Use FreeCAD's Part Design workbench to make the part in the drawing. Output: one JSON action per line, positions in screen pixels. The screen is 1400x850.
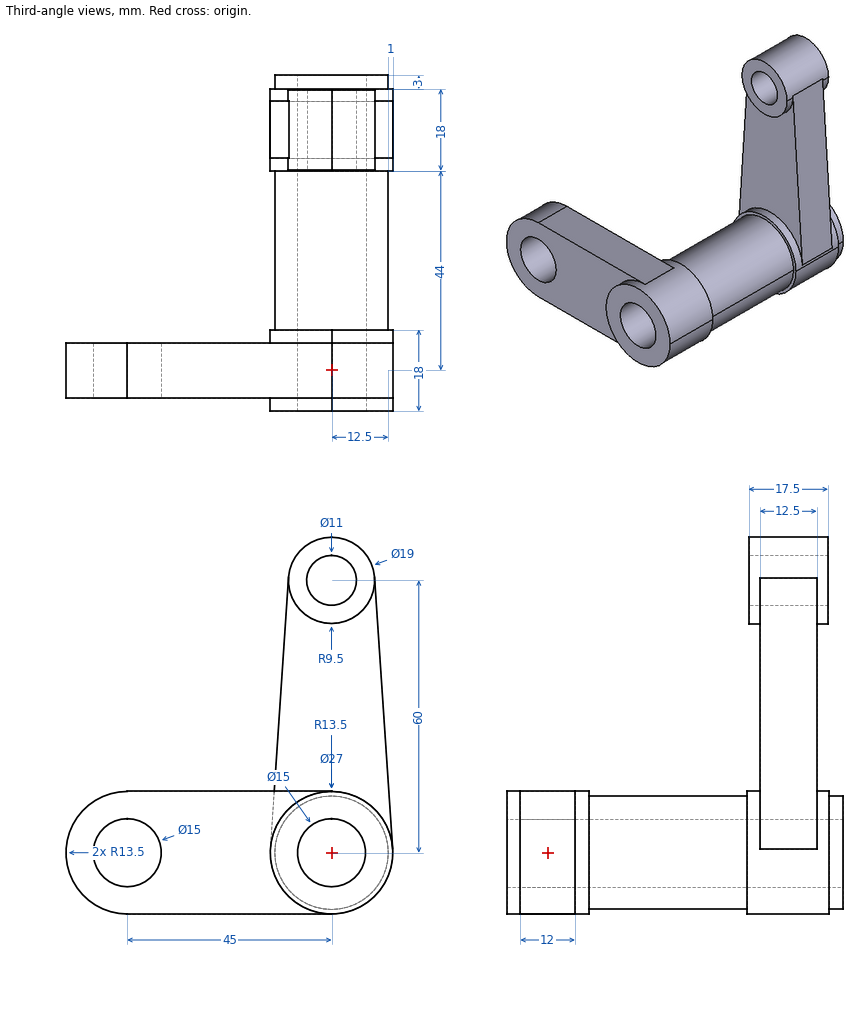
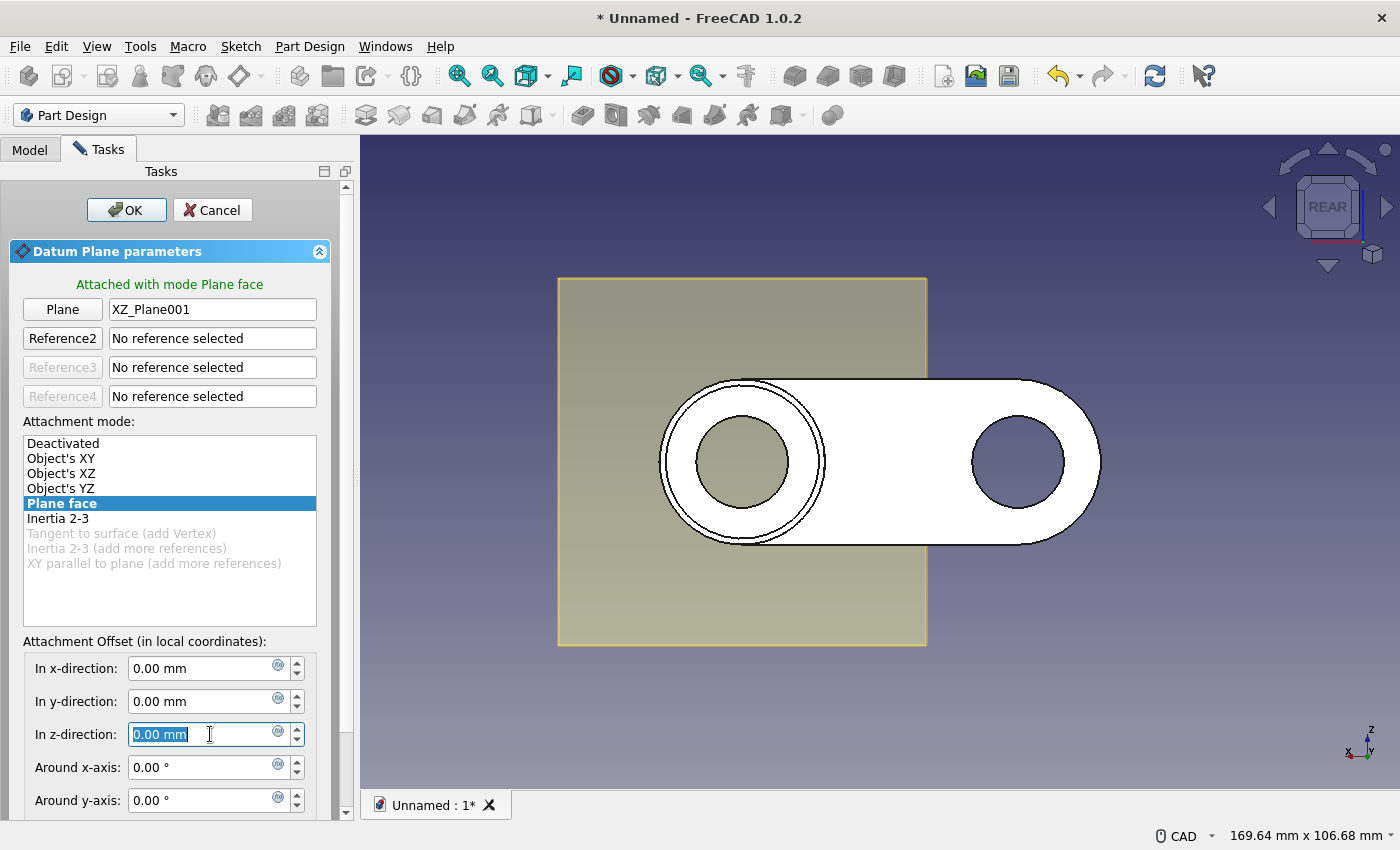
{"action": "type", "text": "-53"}
{"action": "key", "text": "Tab"}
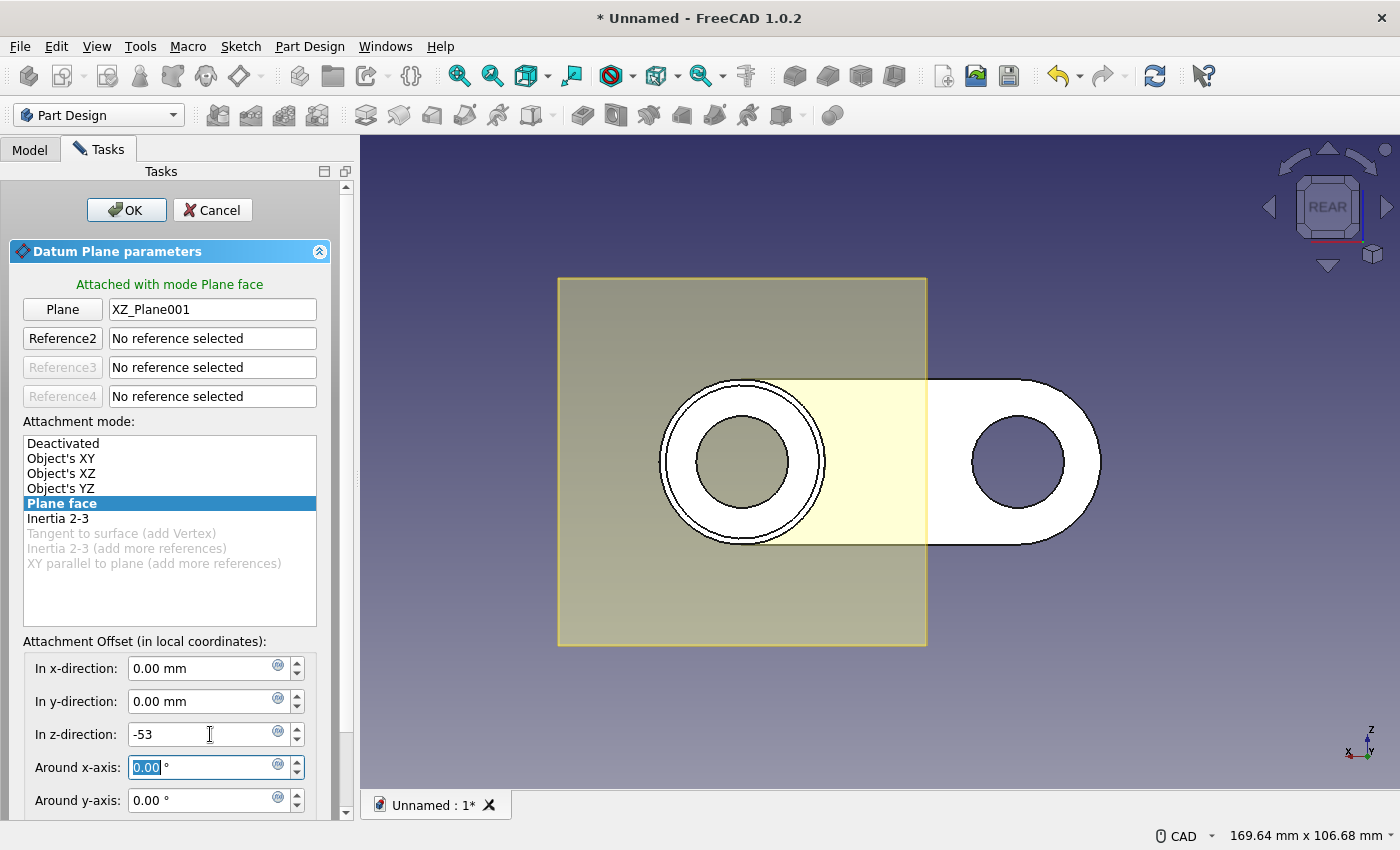
{"action": "left_click", "coordinate": [127, 210]}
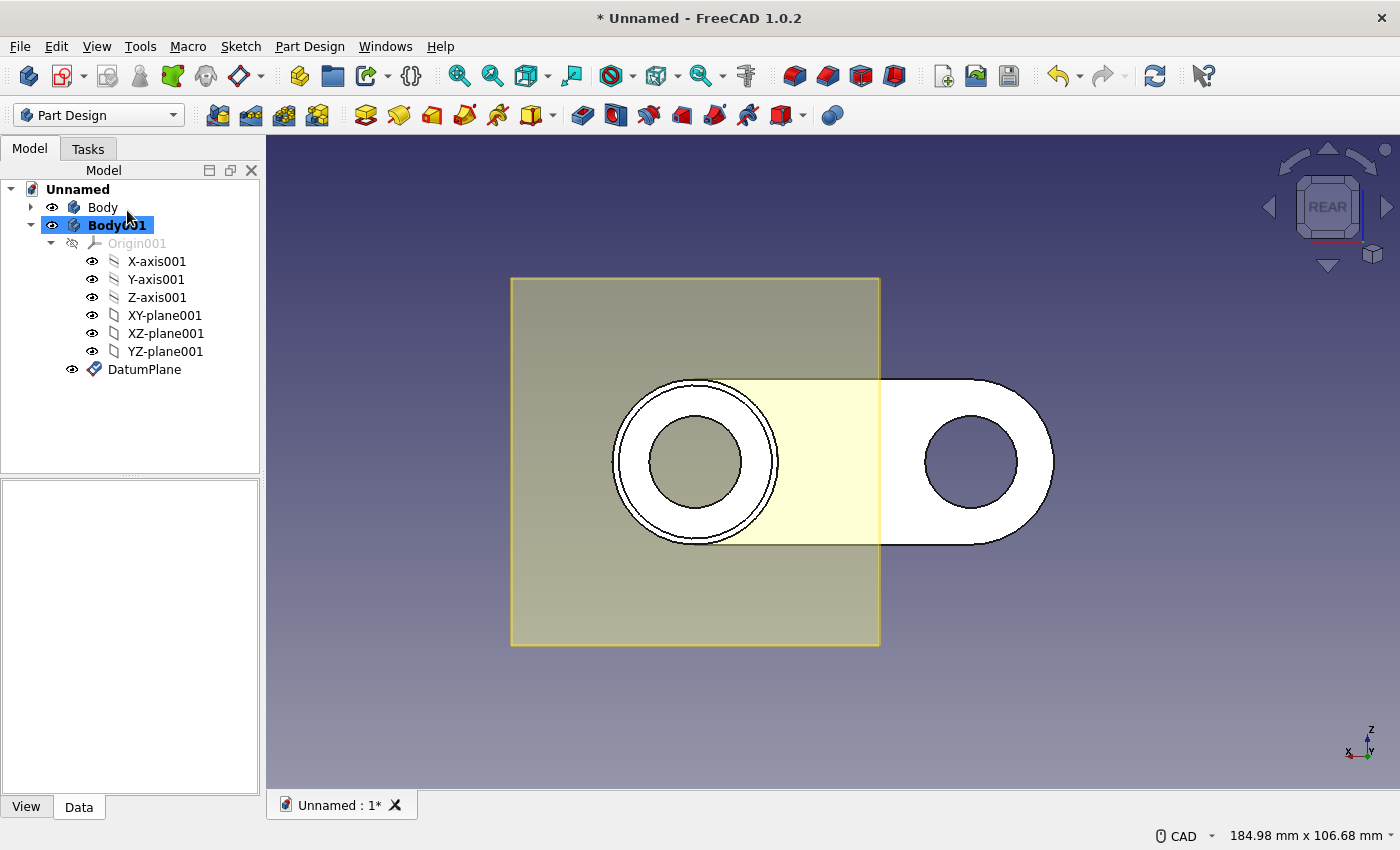
{"action": "left_click", "coordinate": [117, 369]}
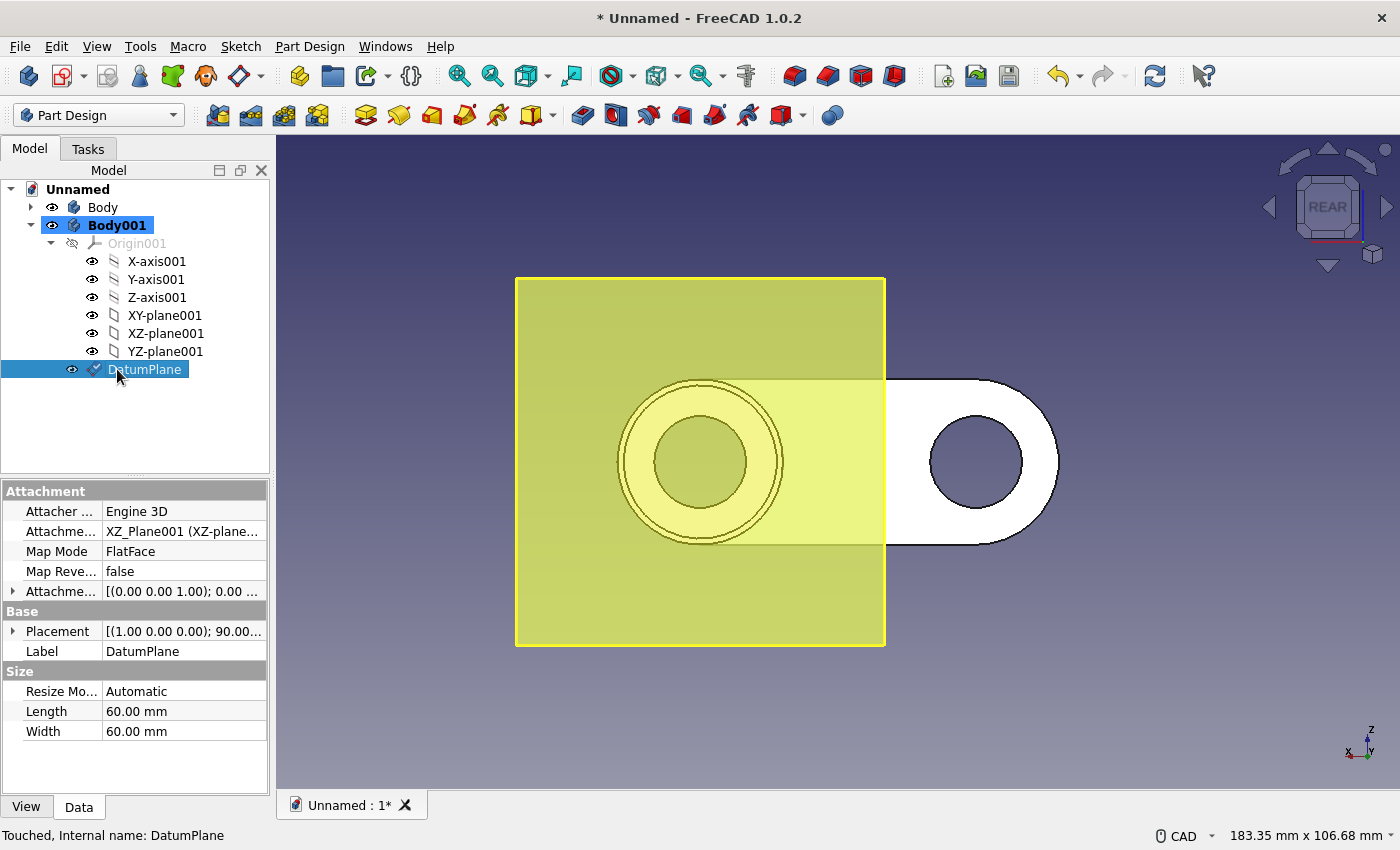
{"action": "left_click", "coordinate": [62, 76]}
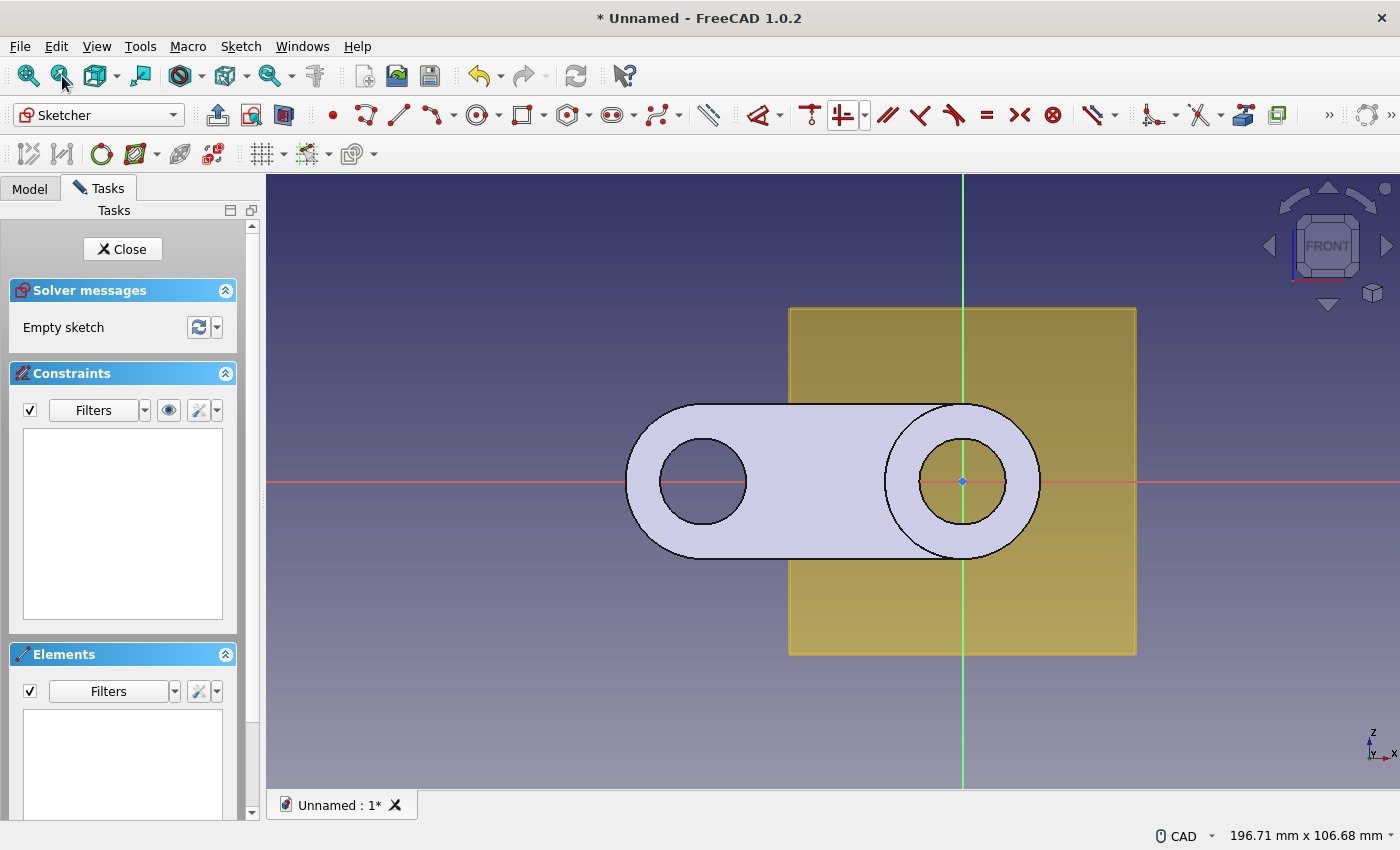
{"action": "scroll", "coordinate": [764, 482], "scroll_direction": "down", "scroll_amount": 5}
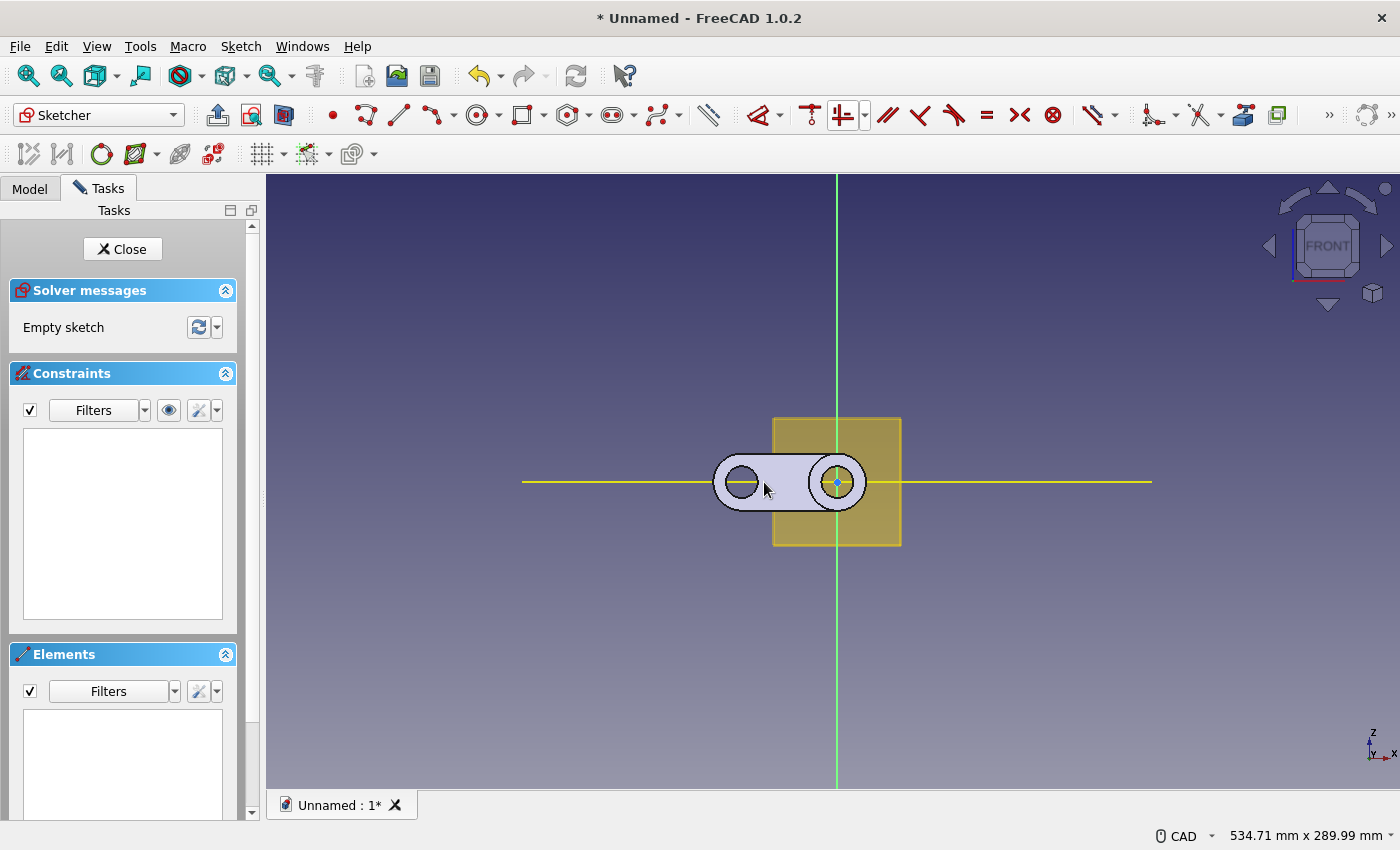
{"action": "scroll", "coordinate": [846, 339], "scroll_direction": "up", "scroll_amount": 11}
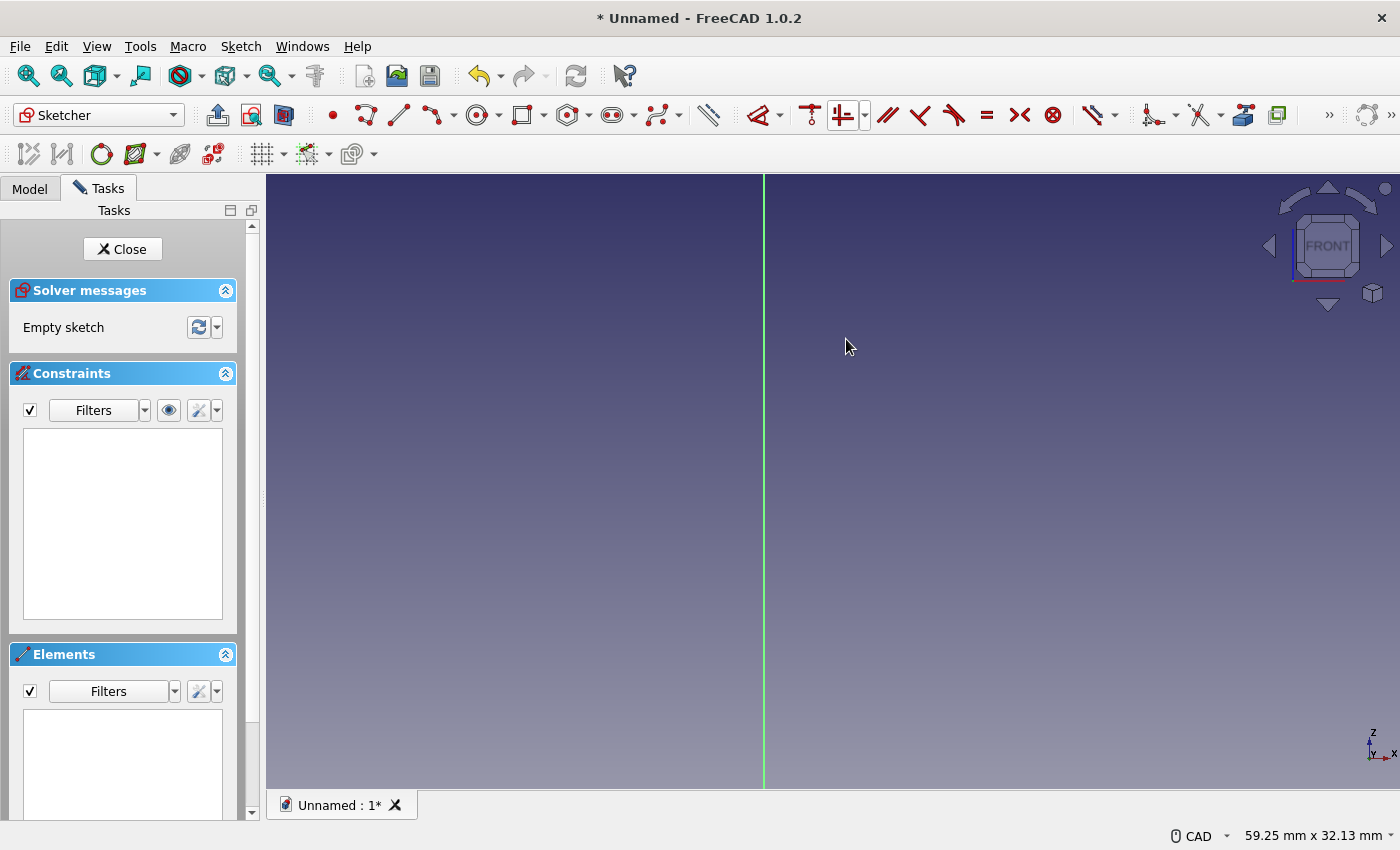
{"action": "key", "text": "g c"}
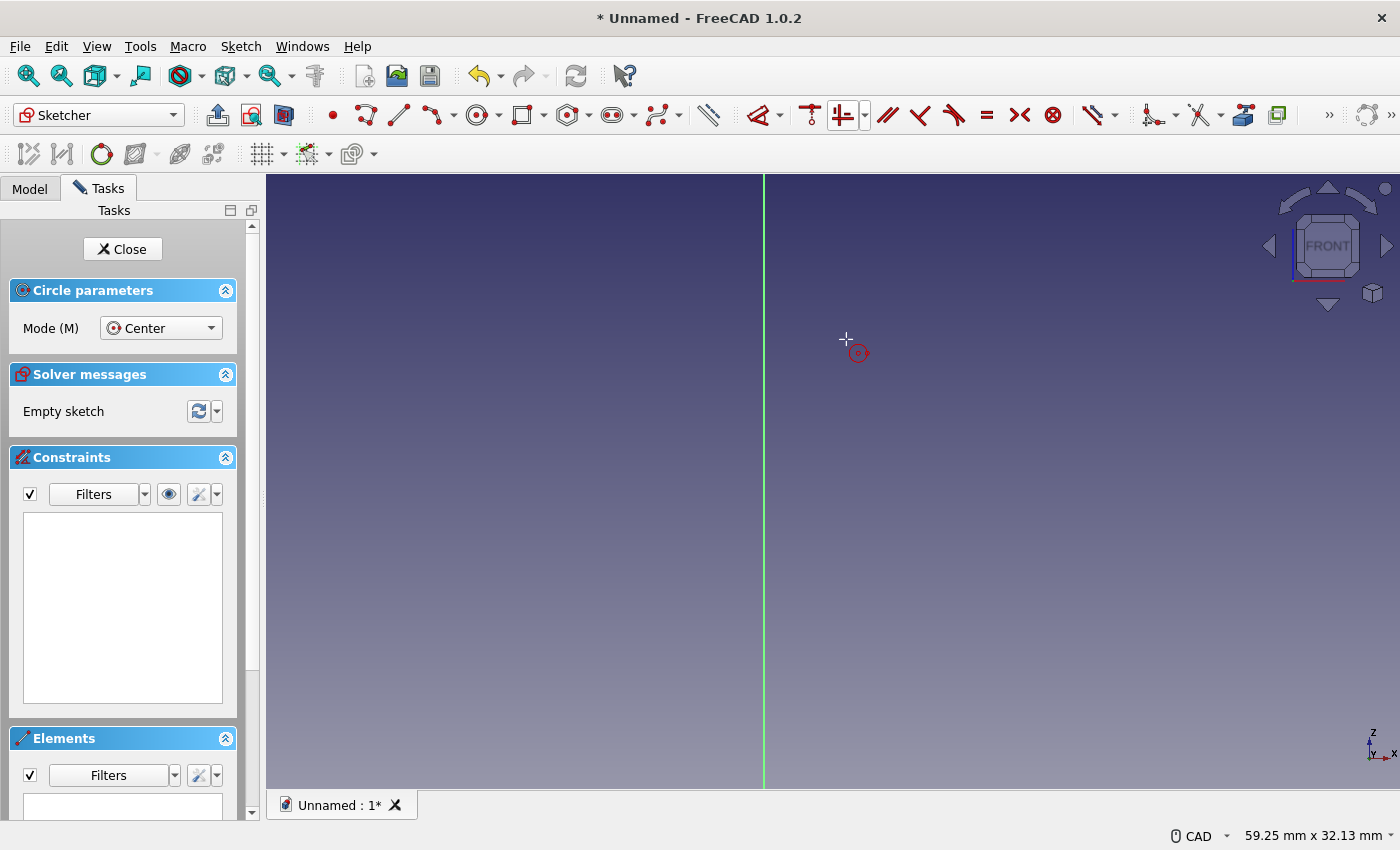
{"action": "left_click", "coordinate": [764, 480]}
{"action": "left_click", "coordinate": [892, 352]}